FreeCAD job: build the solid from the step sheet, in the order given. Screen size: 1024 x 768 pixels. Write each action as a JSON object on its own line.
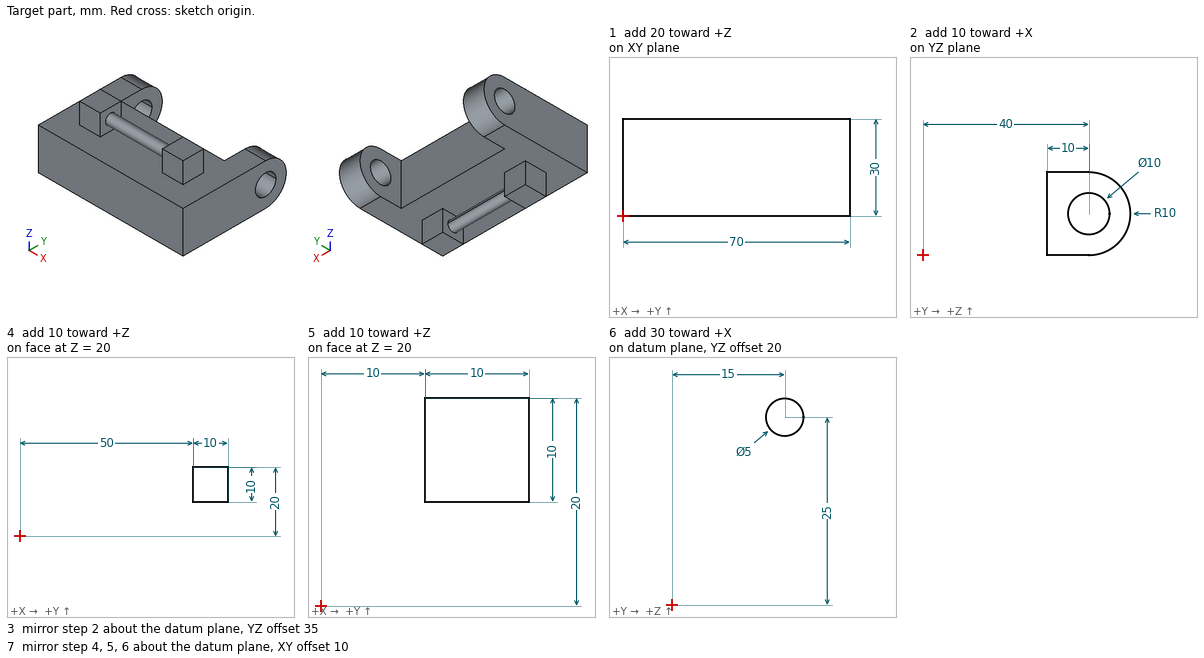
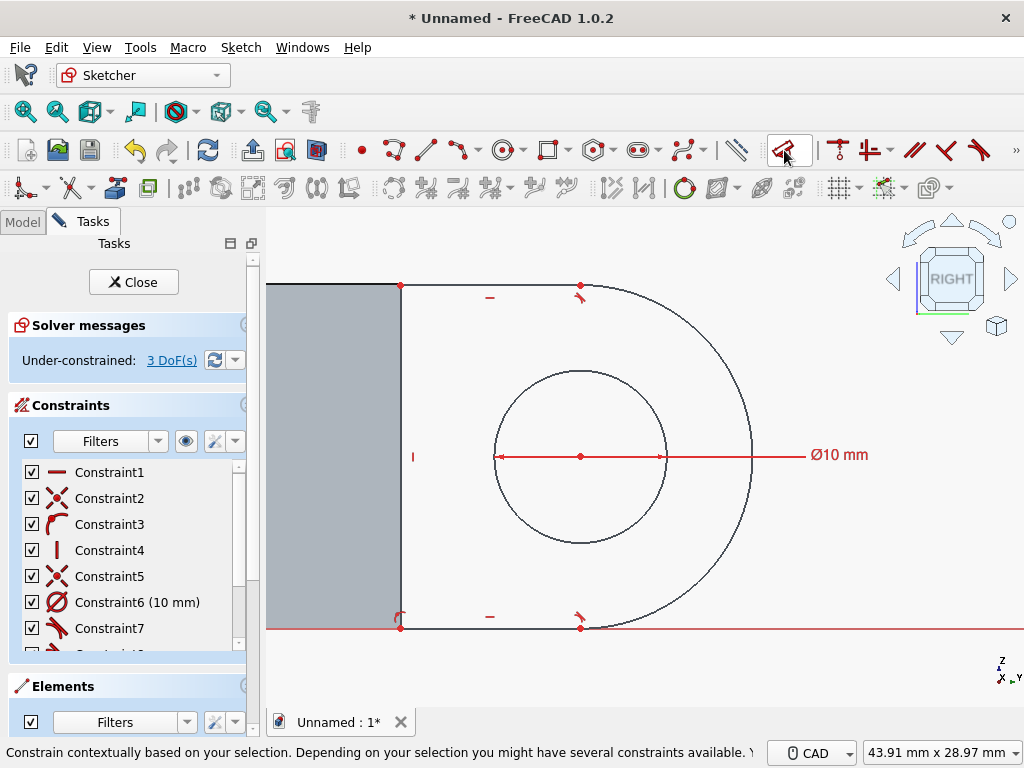
{"action": "left_click", "coordinate": [720, 558]}
{"action": "left_click", "coordinate": [746, 577]}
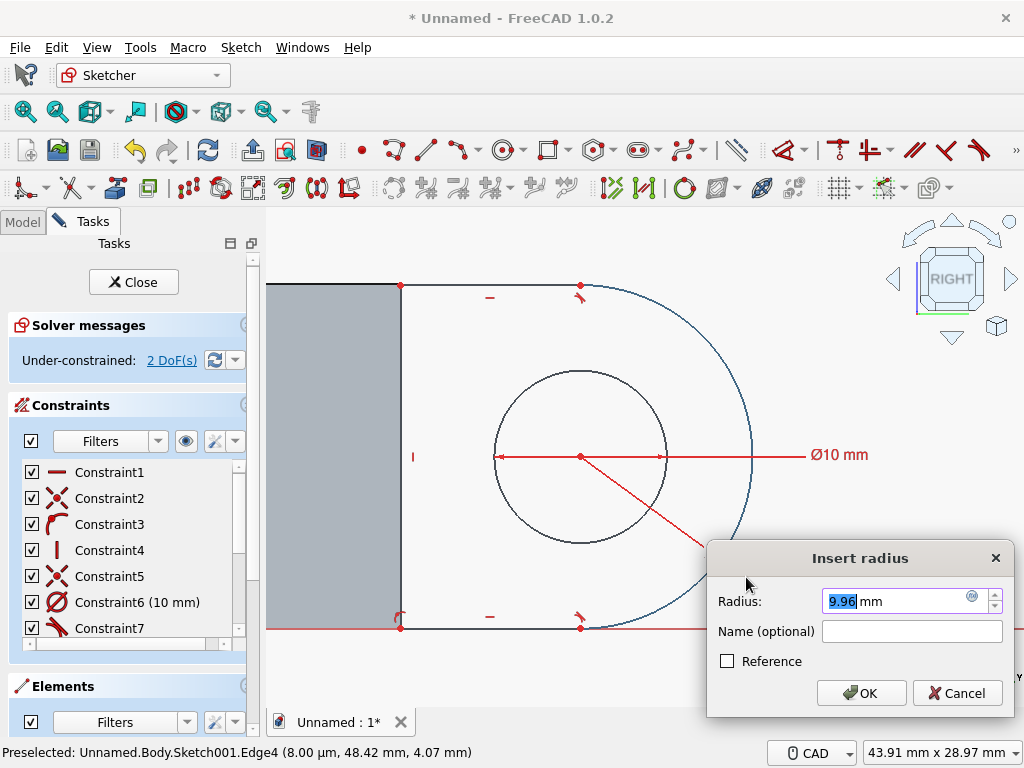
{"action": "type", "text": "10"}
{"action": "key", "text": "Return"}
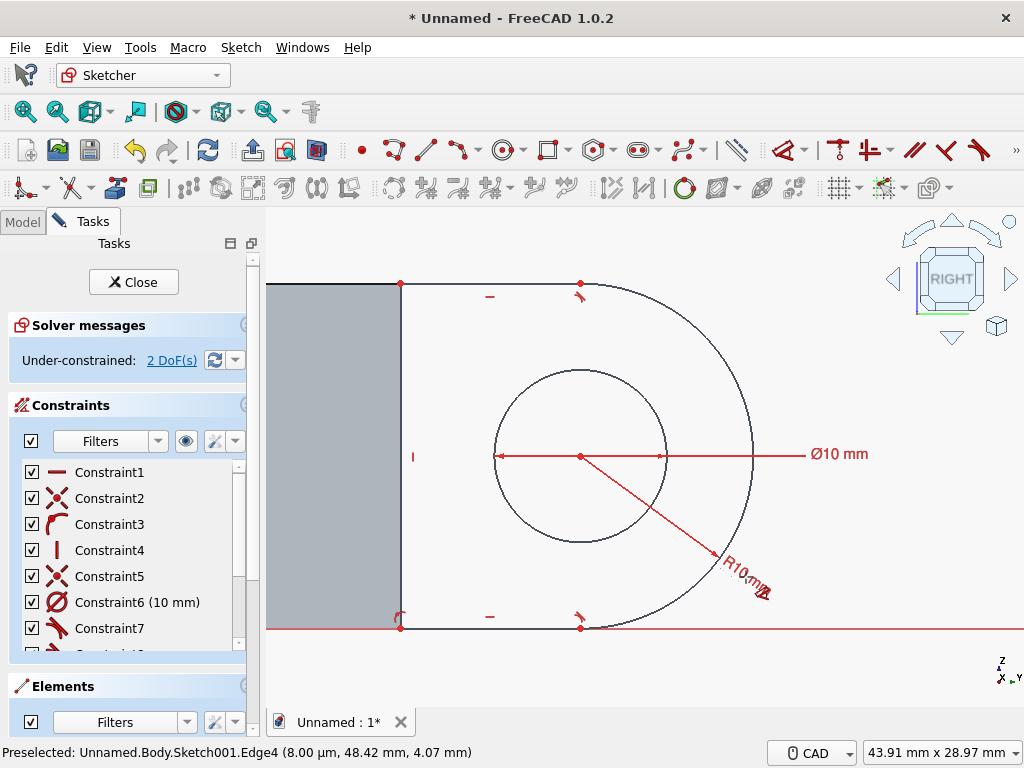
{"action": "left_click", "coordinate": [527, 284]}
{"action": "left_click", "coordinate": [491, 250]}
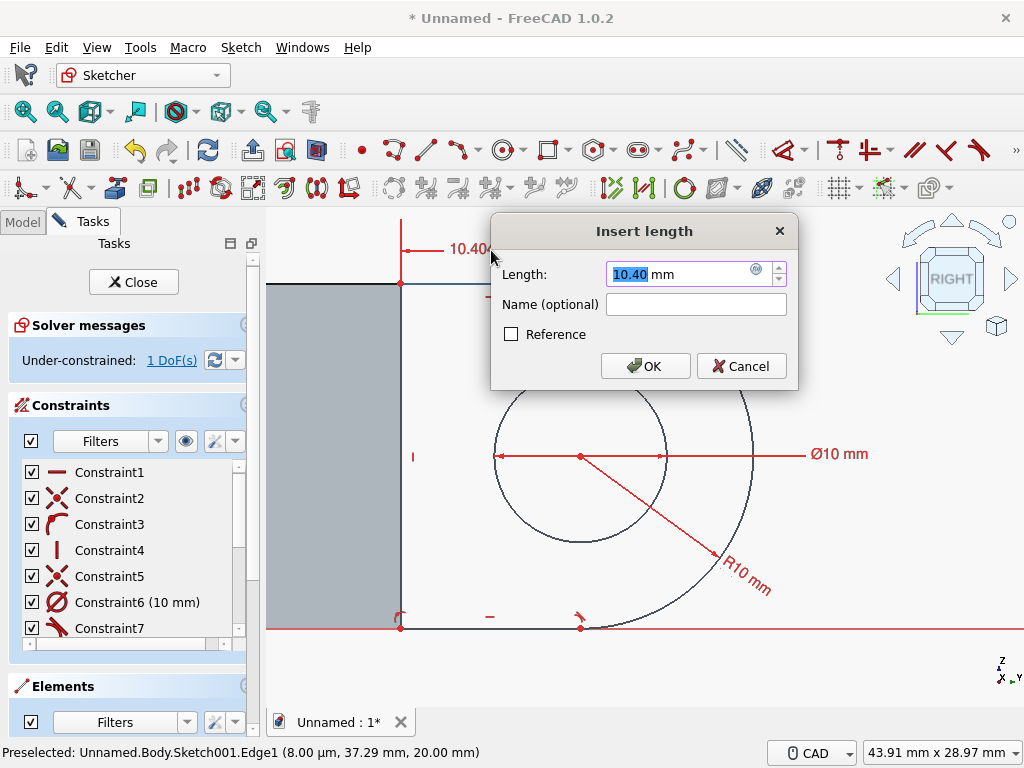
{"action": "type", "text": "10"}
{"action": "key", "text": "Return"}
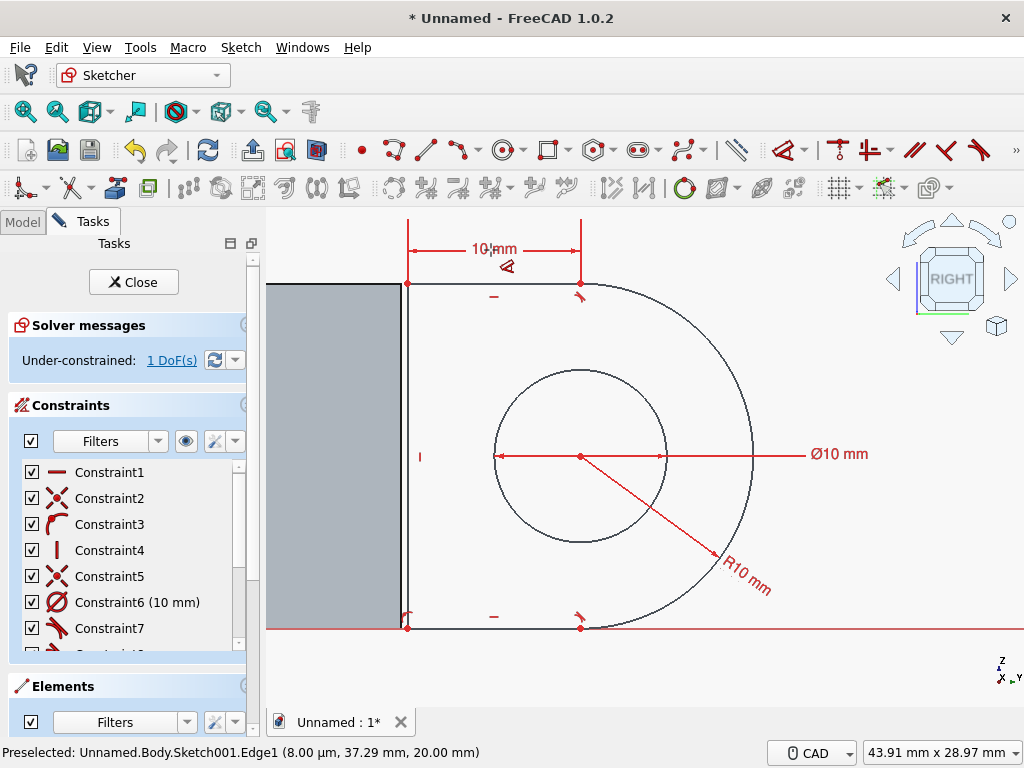
{"action": "left_click", "coordinate": [581, 456]}
{"action": "left_click", "coordinate": [437, 663]}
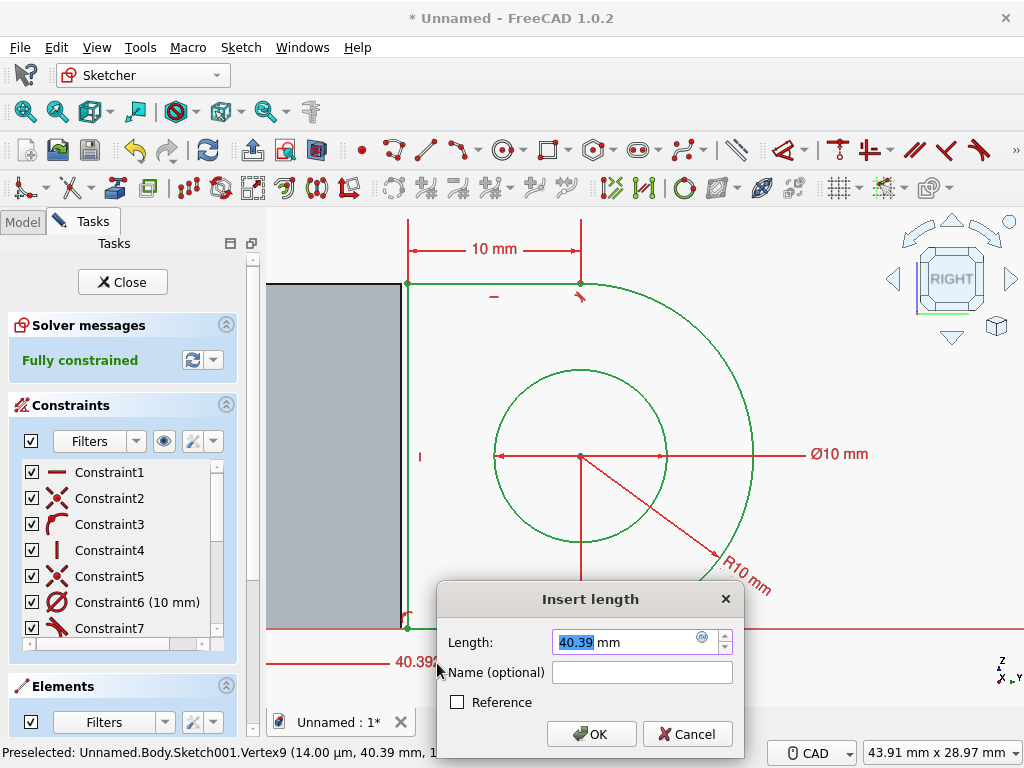
{"action": "type", "text": "40"}
{"action": "key", "text": "Return"}
{"action": "key", "text": "Escape"}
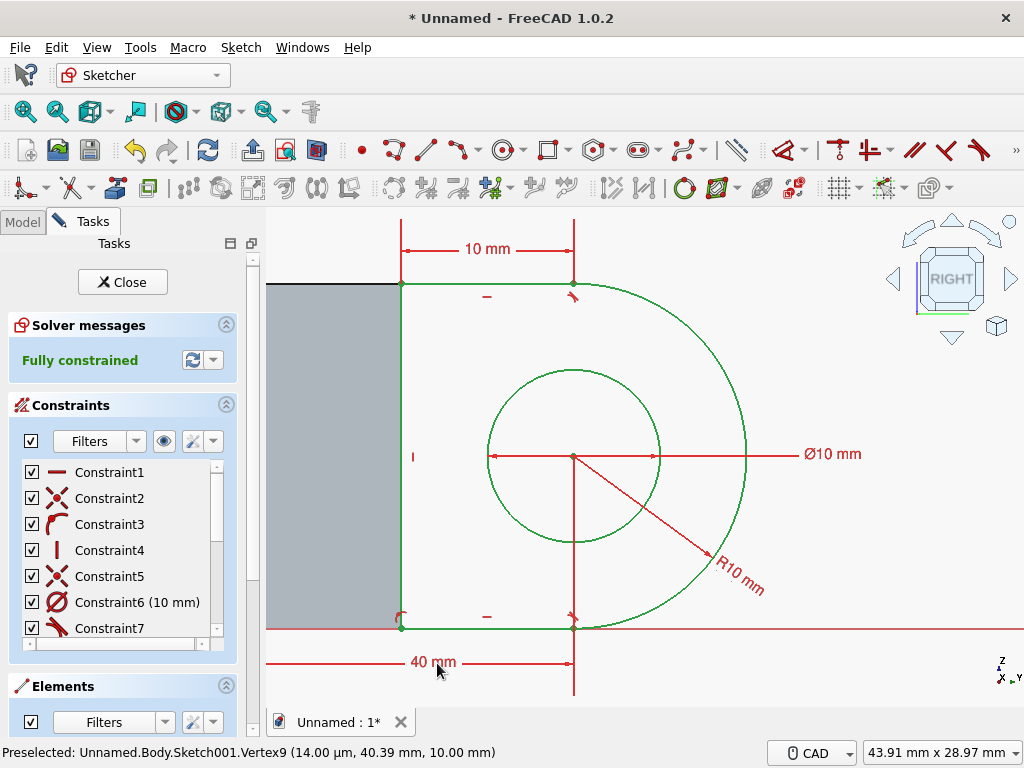
{"action": "left_click", "coordinate": [123, 282]}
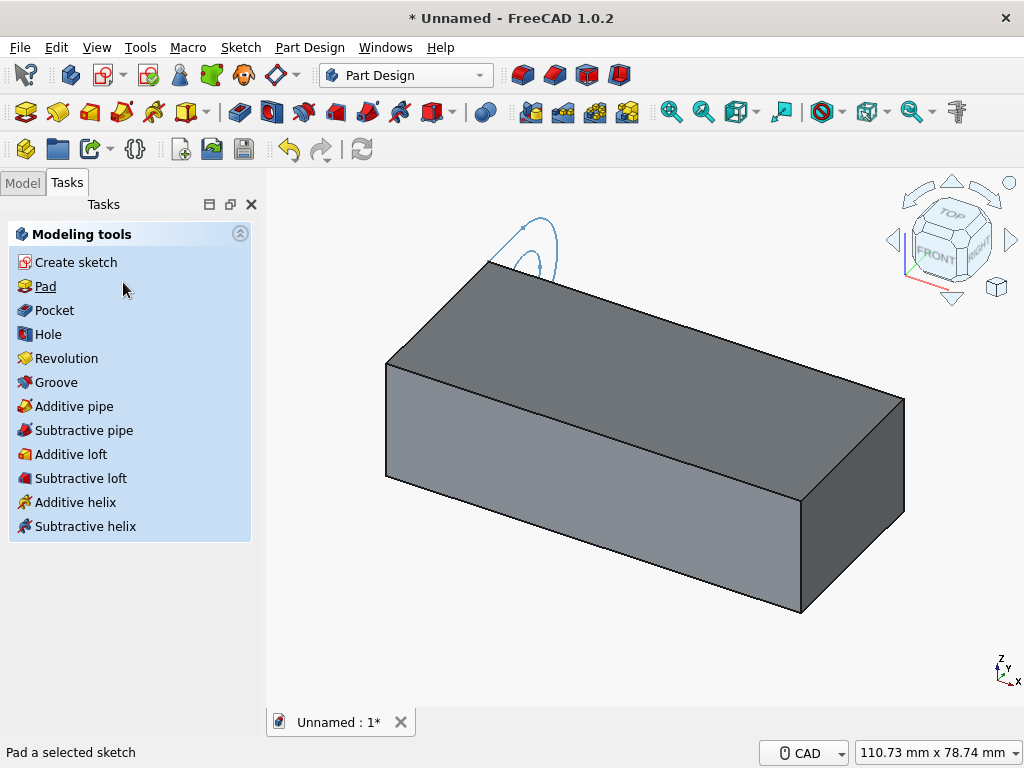
{"action": "left_click", "coordinate": [26, 112]}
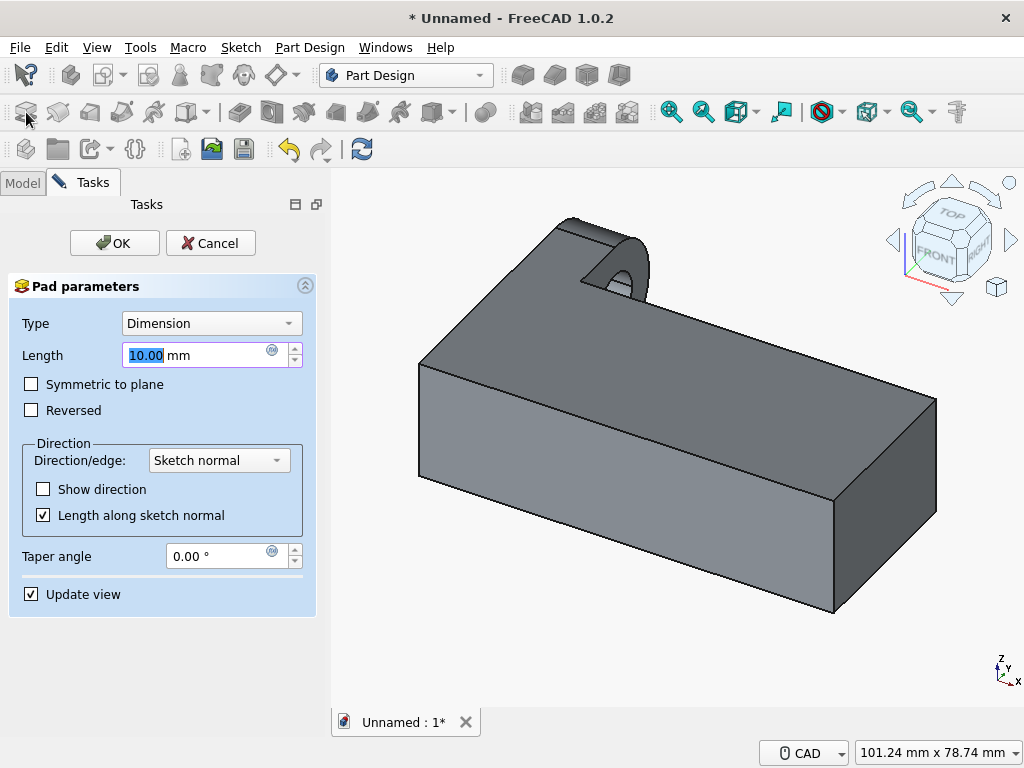
{"action": "type", "text": "10"}
{"action": "key", "text": "Tab"}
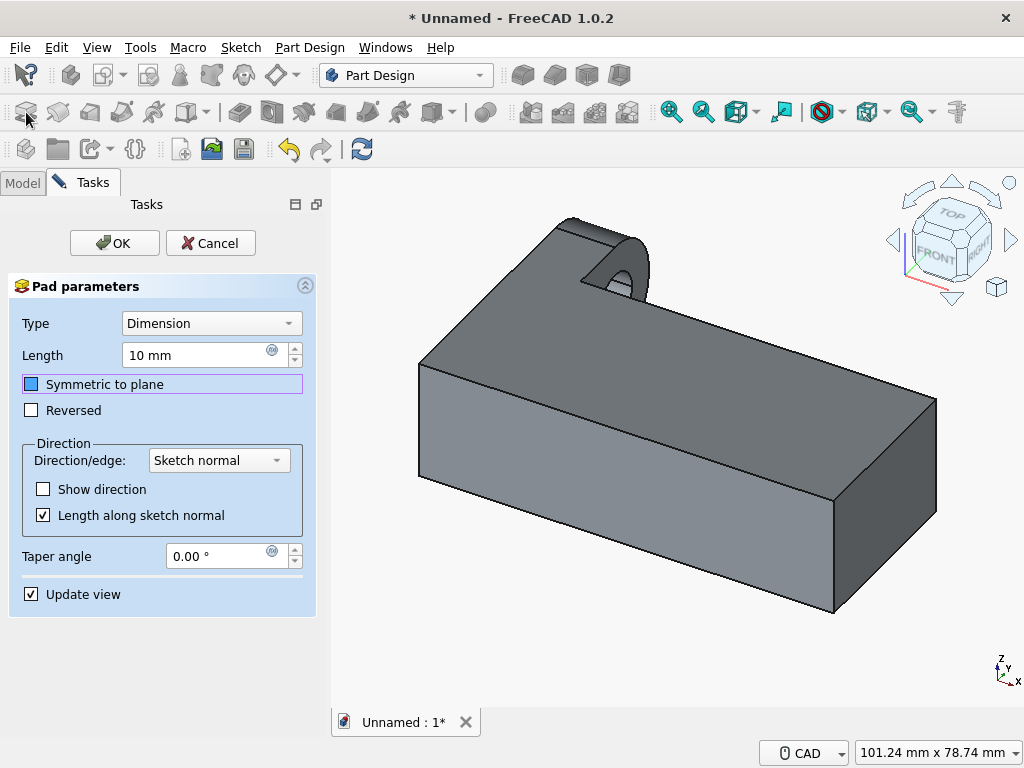
{"action": "left_click", "coordinate": [115, 243]}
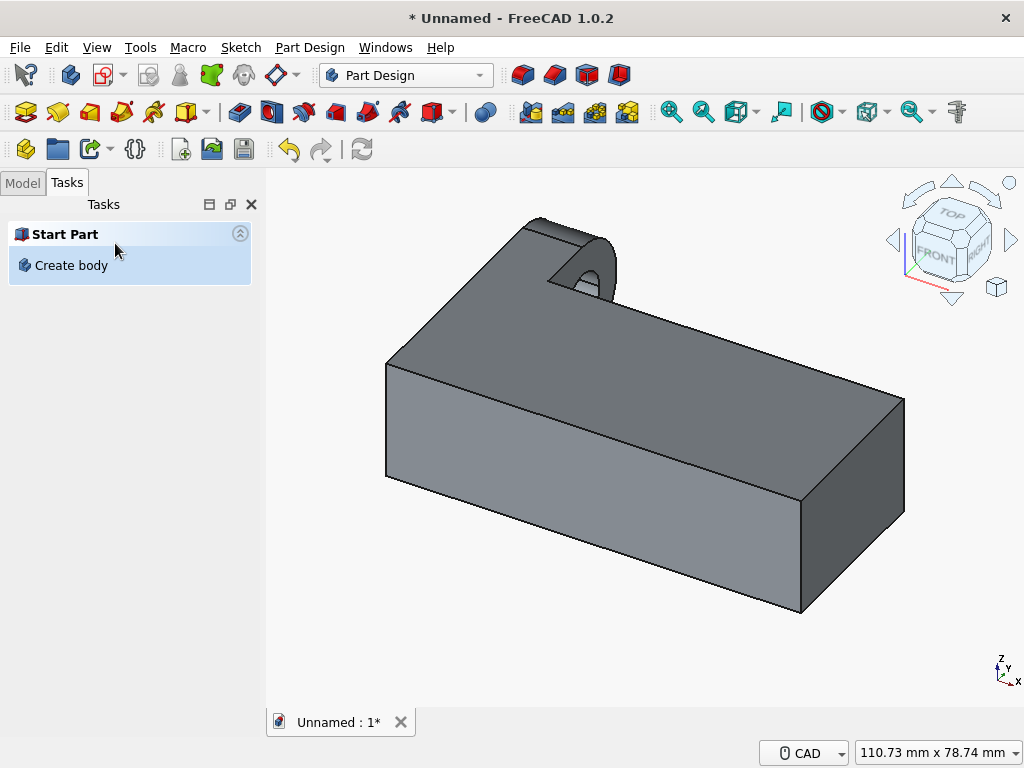
{"action": "left_click", "coordinate": [23, 182]}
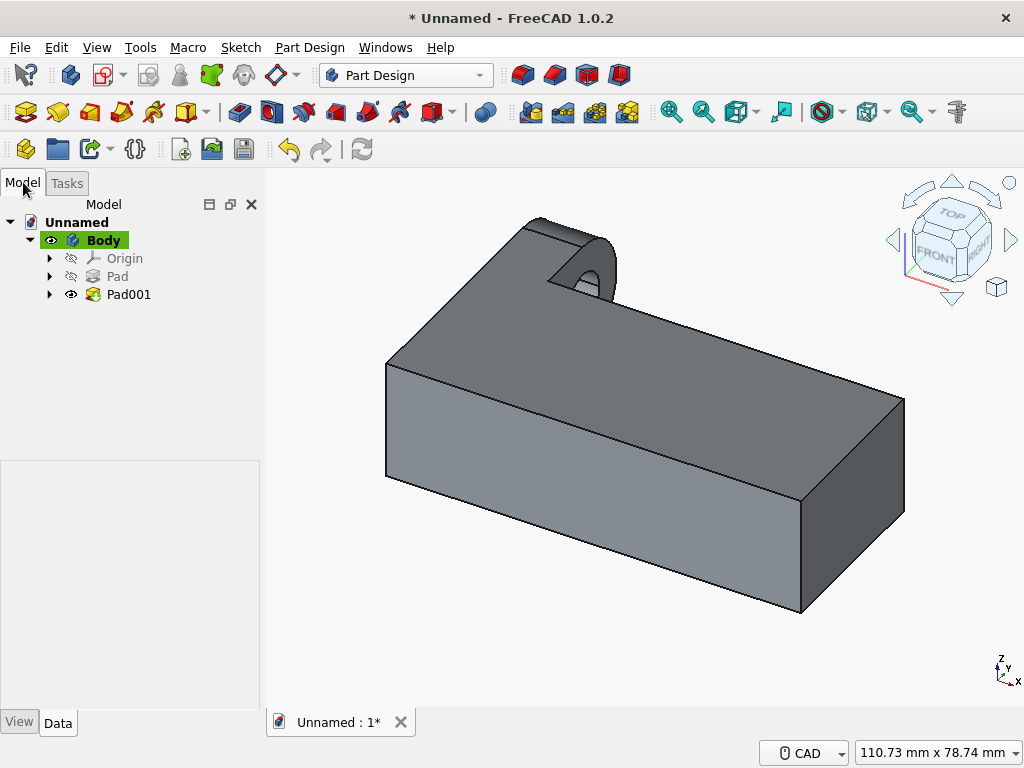
{"action": "left_click", "coordinate": [50, 258]}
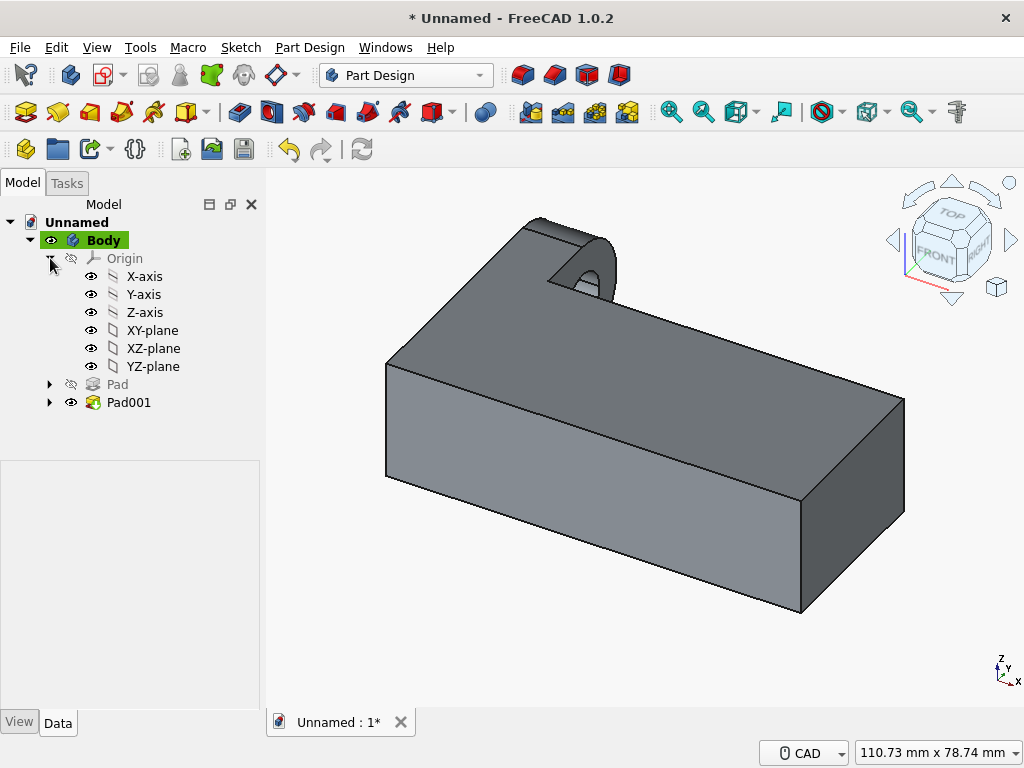
{"action": "left_click", "coordinate": [136, 366]}